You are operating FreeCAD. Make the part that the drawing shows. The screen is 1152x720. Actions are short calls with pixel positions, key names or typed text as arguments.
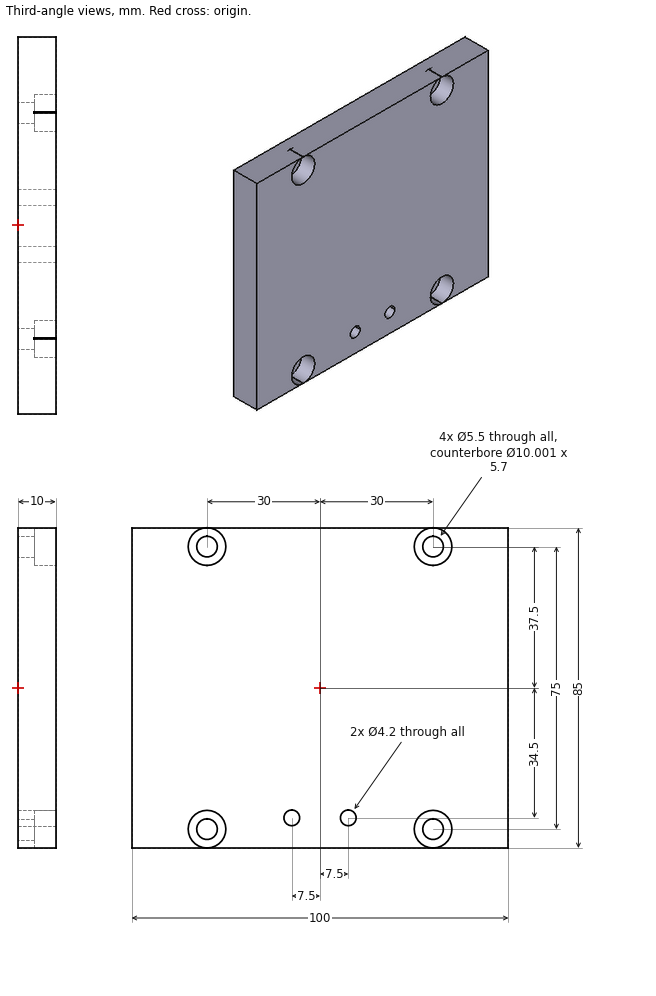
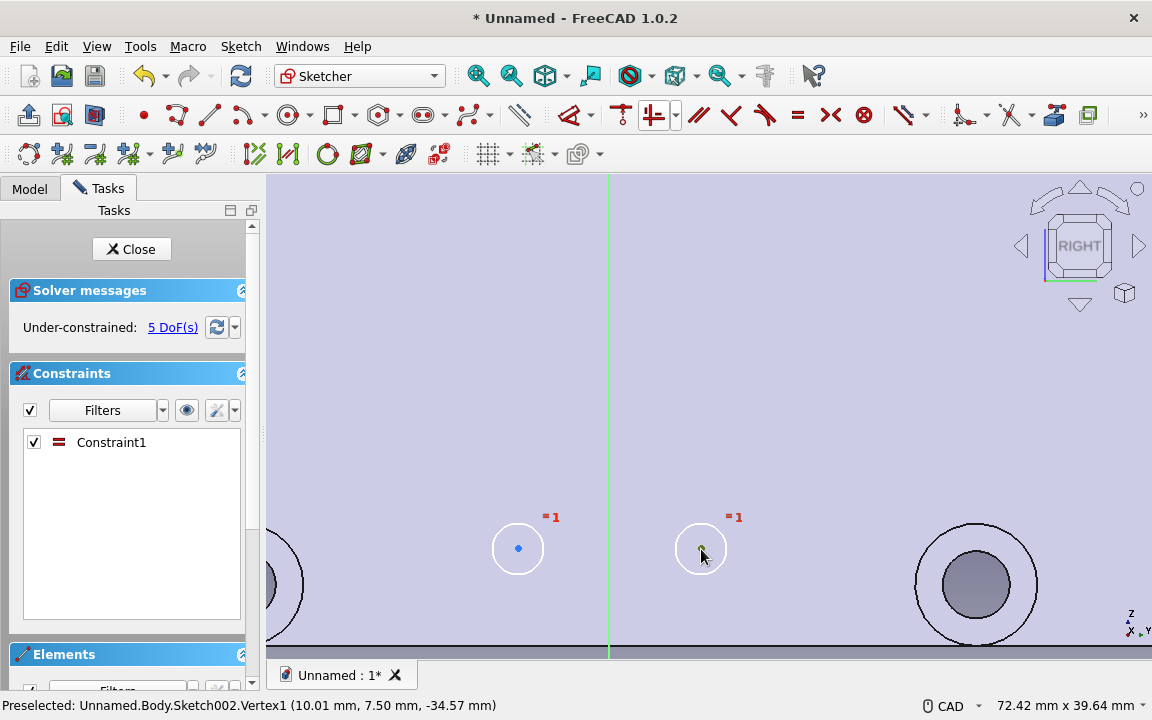
click(518, 549)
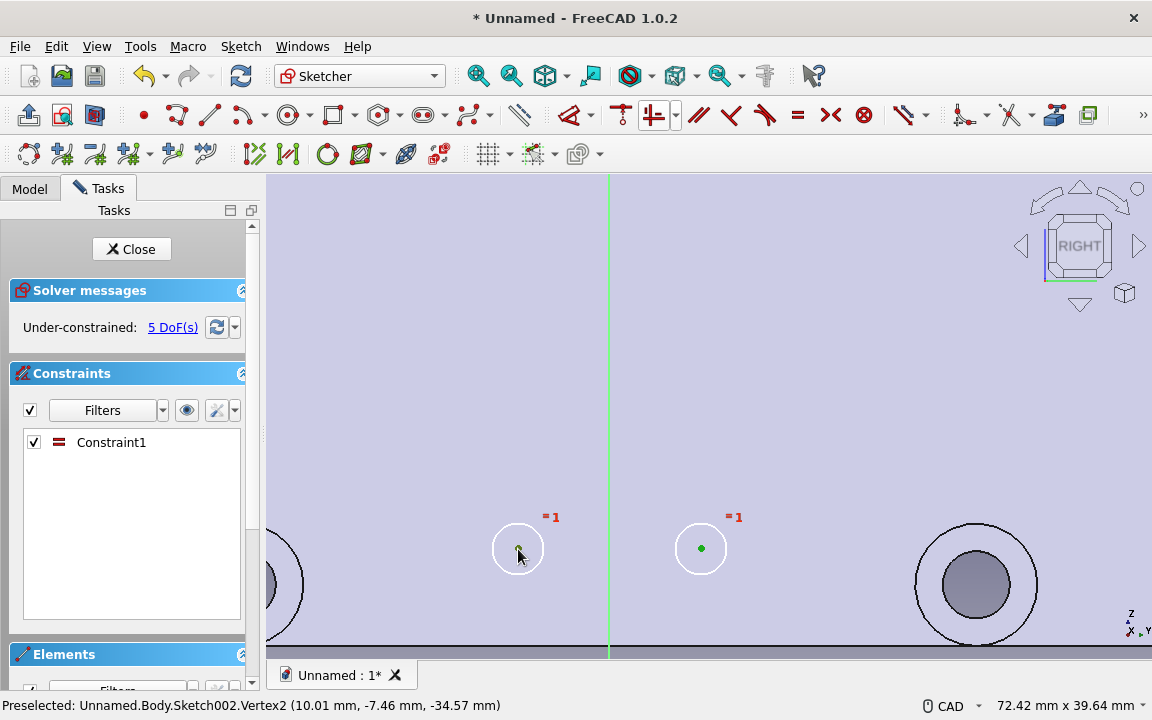
click(676, 116)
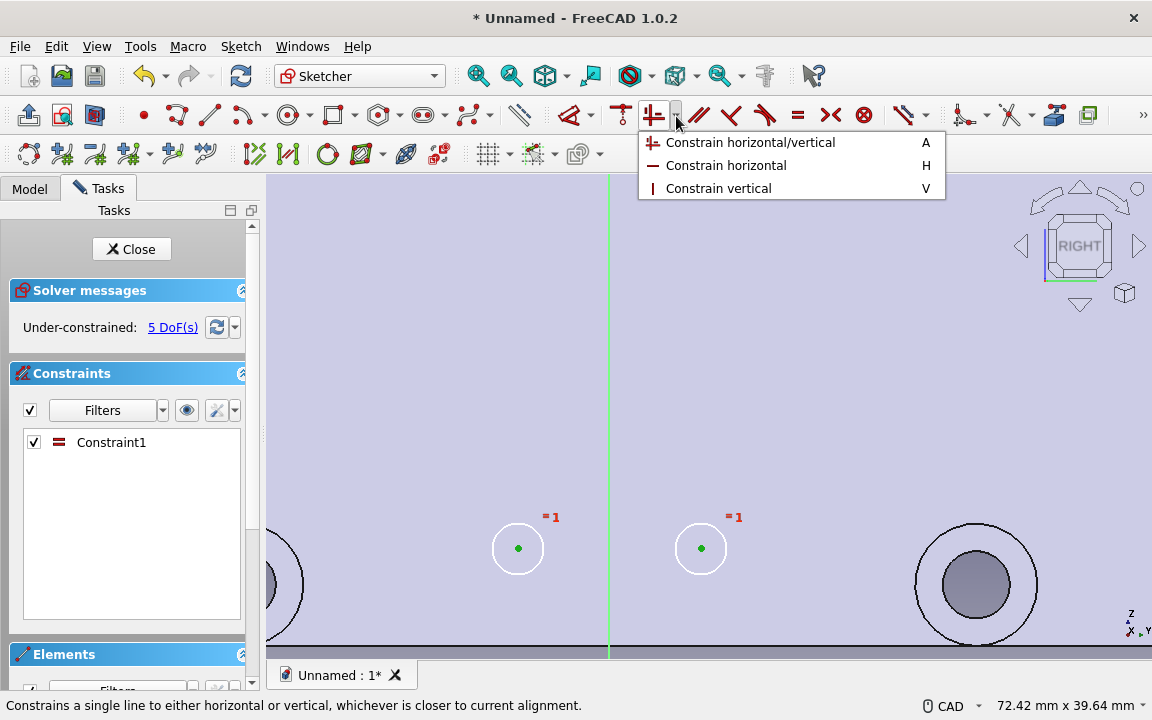
click(792, 166)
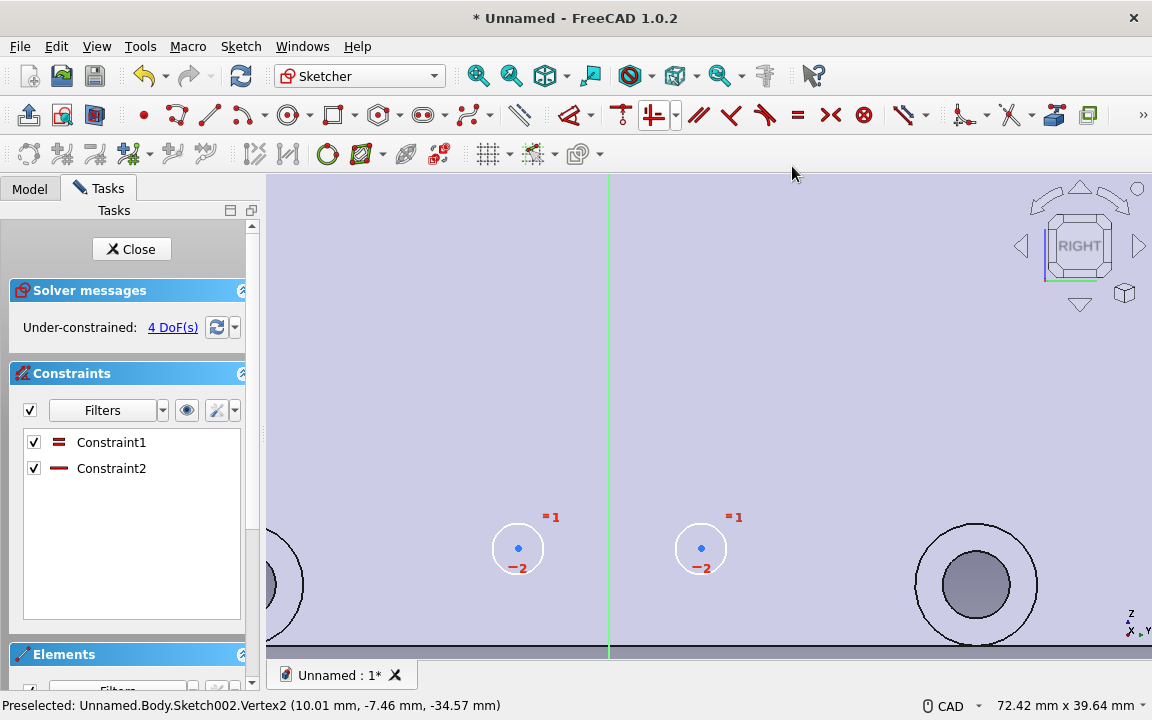
click(568, 116)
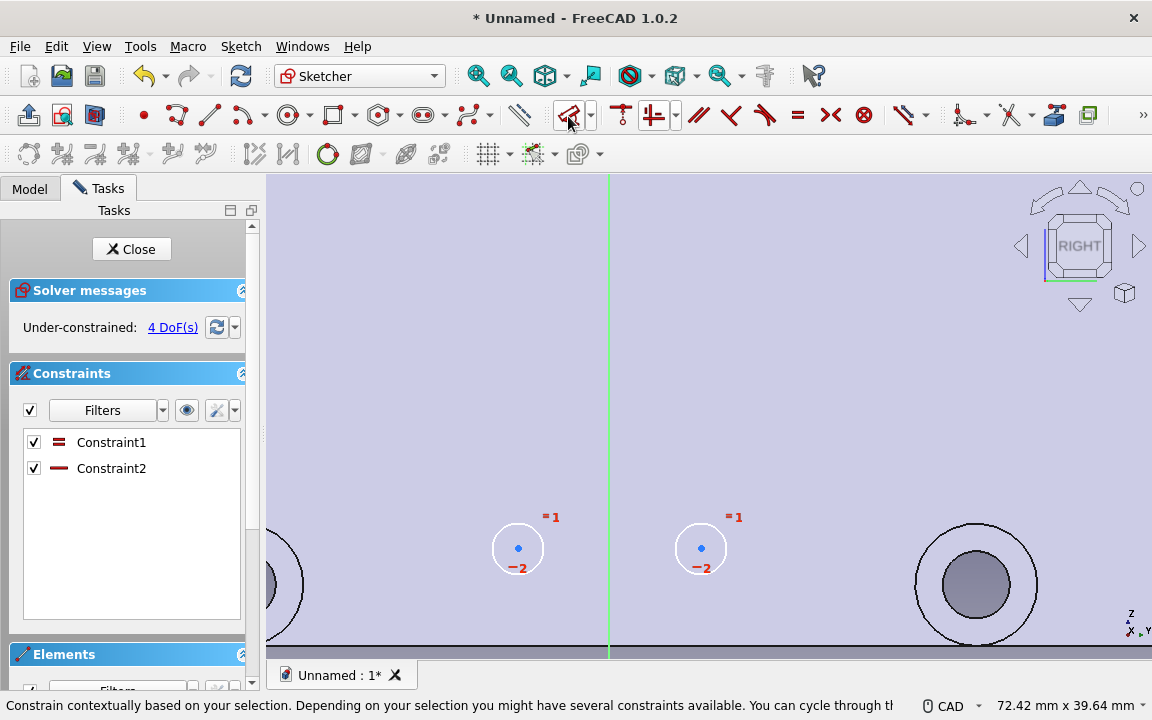
click(719, 531)
click(742, 508)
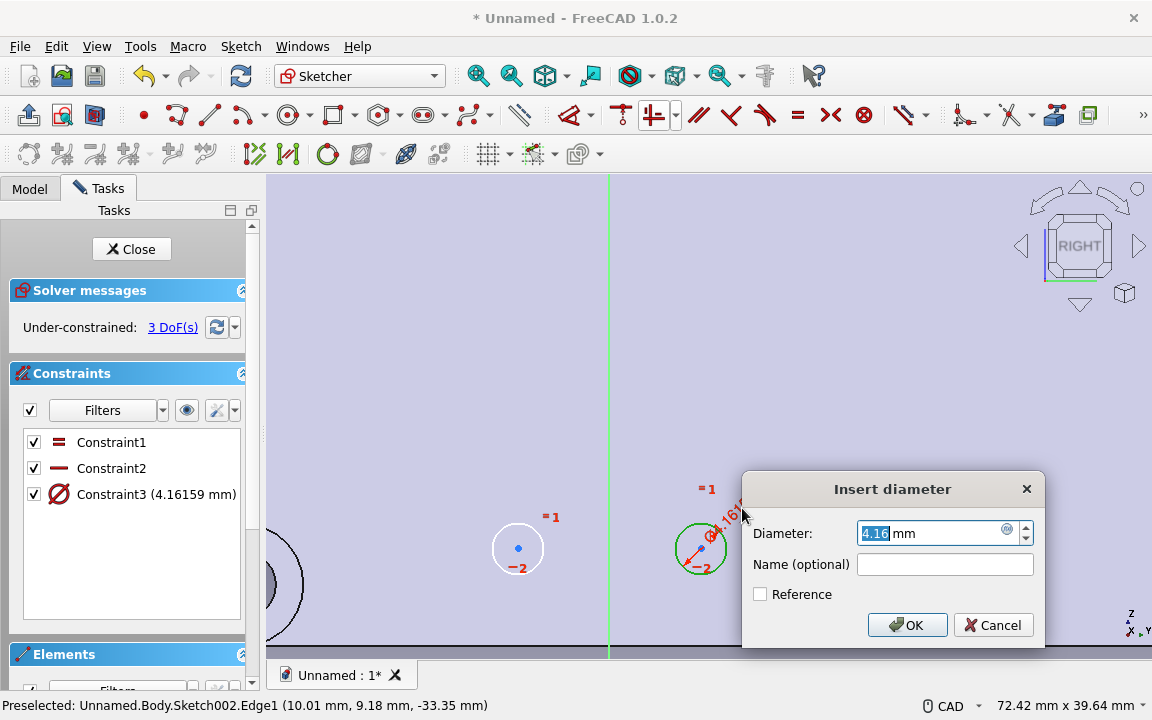
text(4.2)
key(Return)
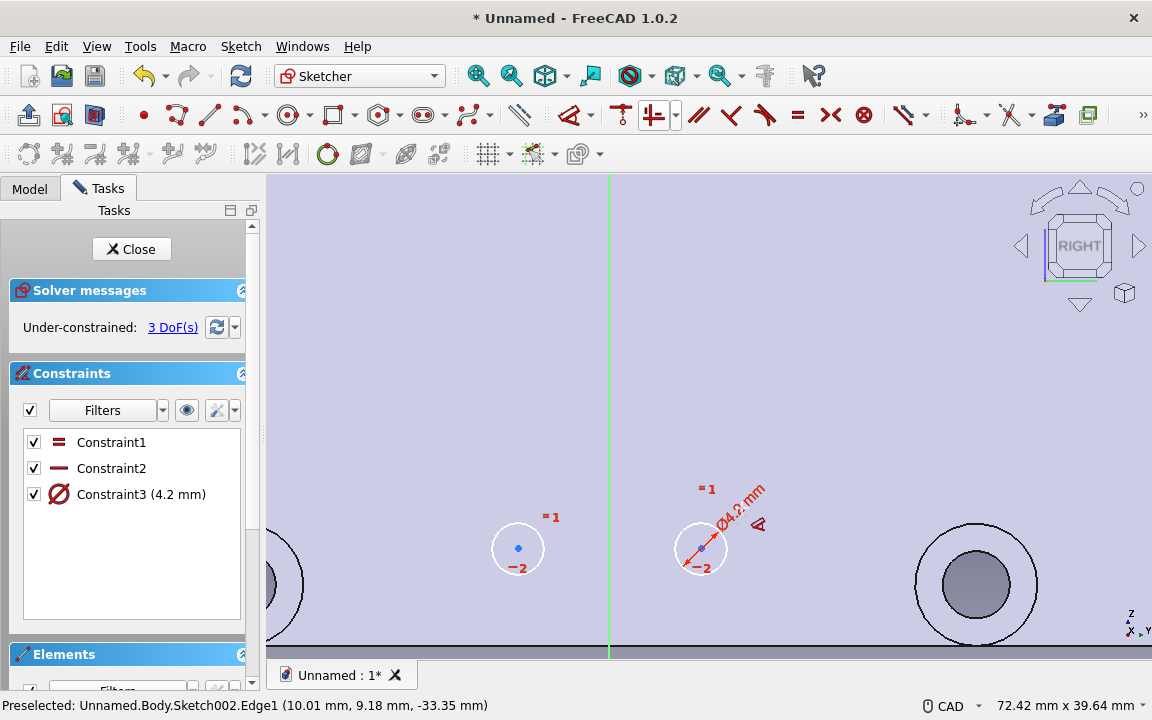
click(701, 549)
click(655, 583)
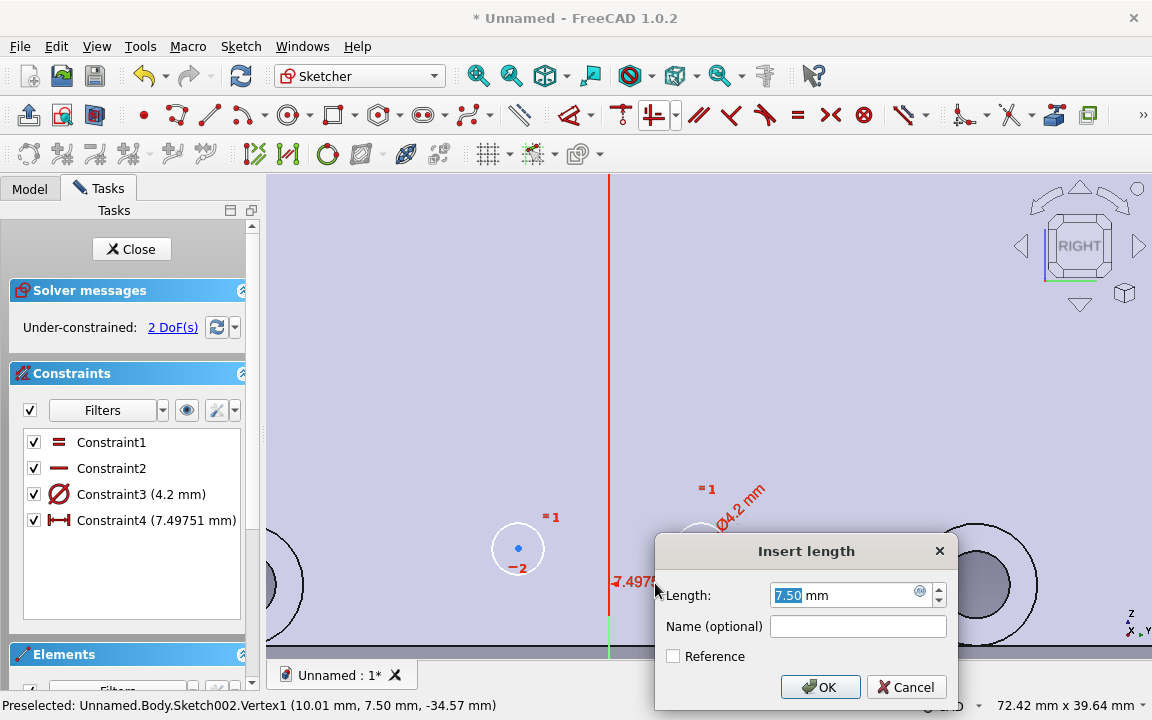
text(7.5)
key(Return)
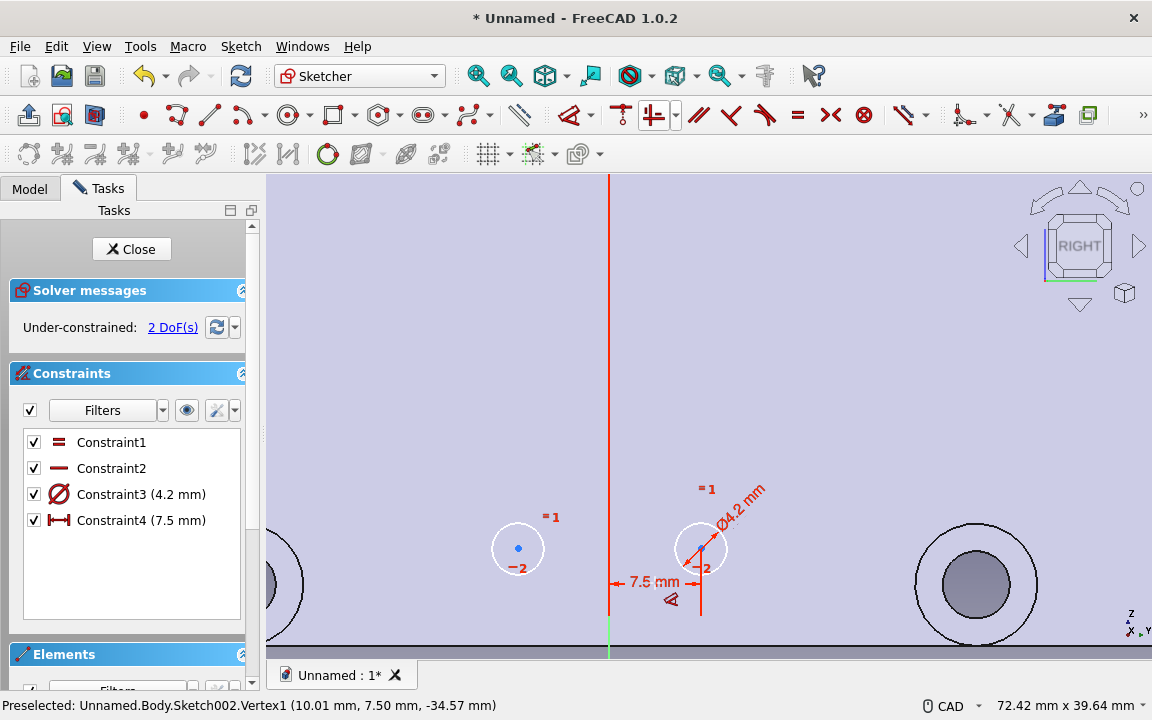
click(518, 549)
click(564, 583)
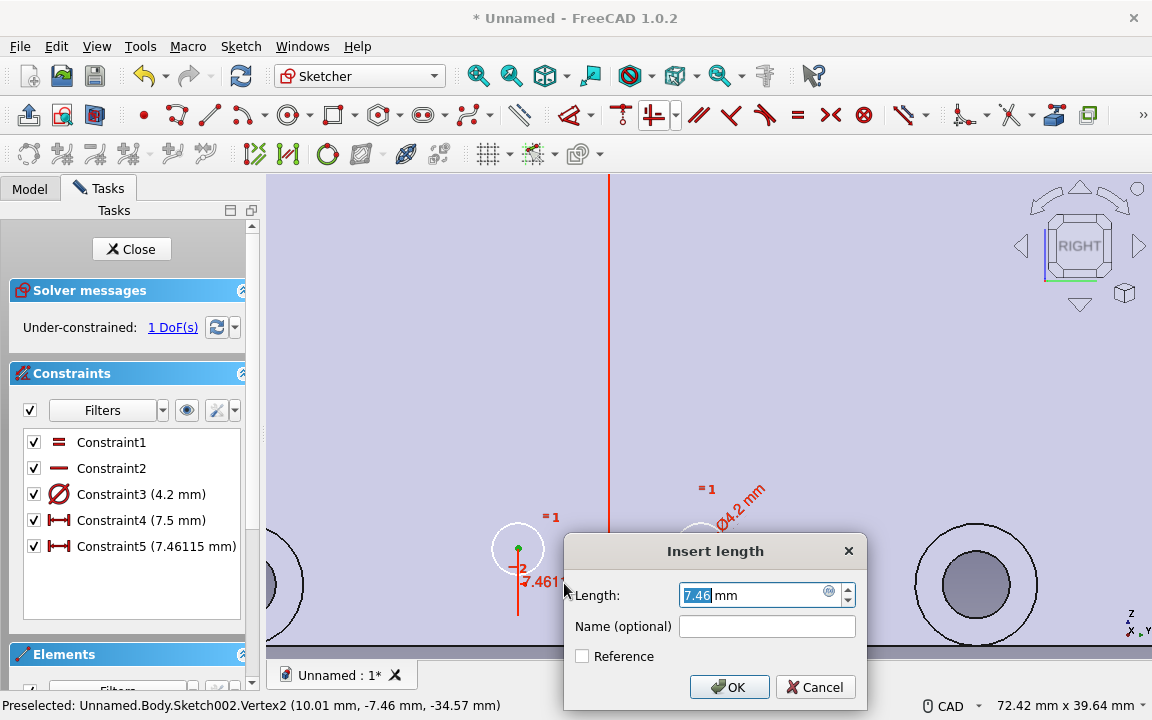
text(7.5)
key(Return)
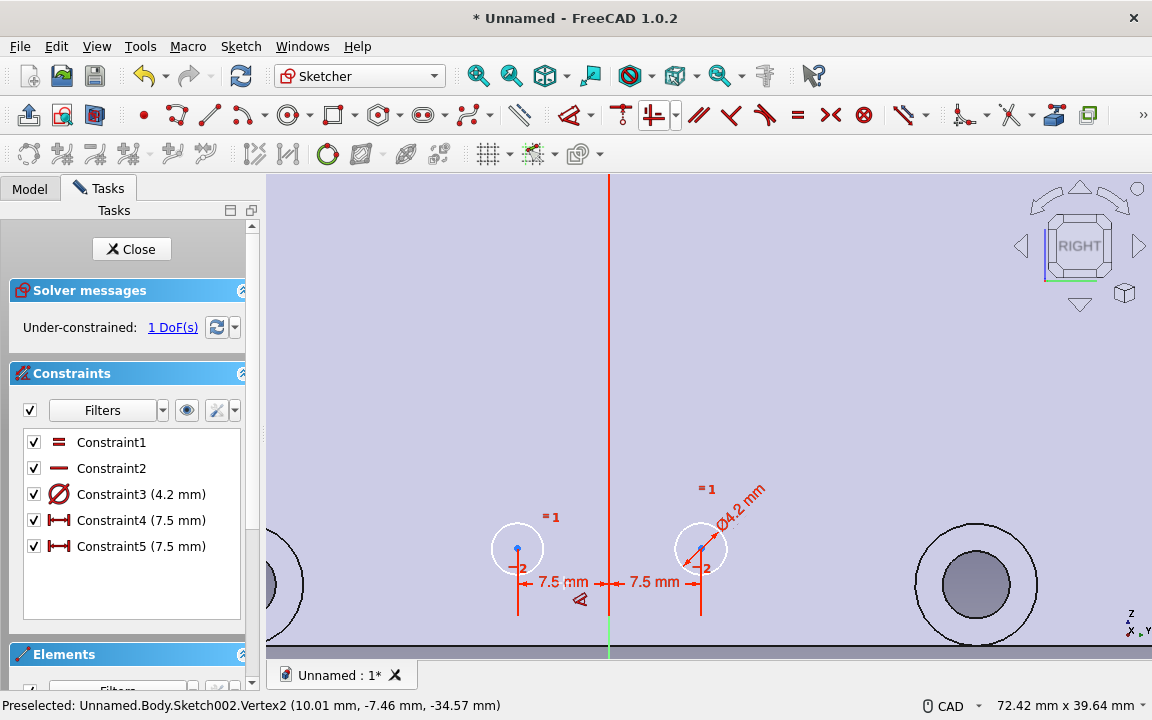
click(701, 549)
click(735, 375)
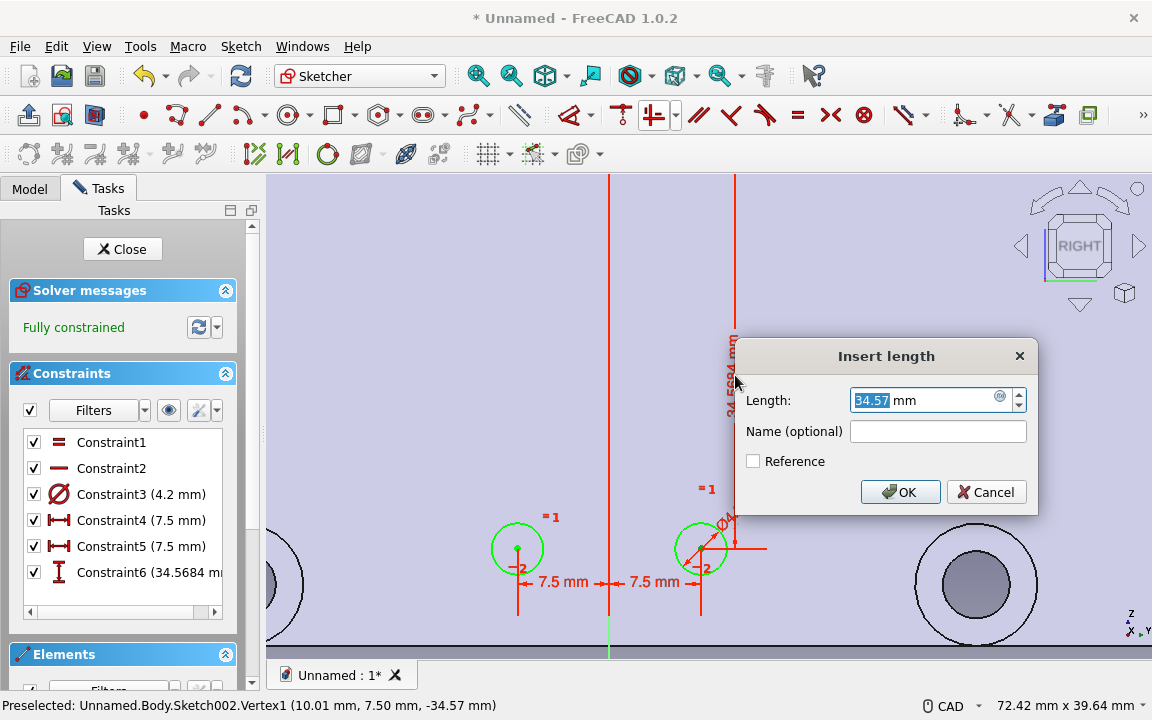
text(34.5)
key(Return)
key(Escape)